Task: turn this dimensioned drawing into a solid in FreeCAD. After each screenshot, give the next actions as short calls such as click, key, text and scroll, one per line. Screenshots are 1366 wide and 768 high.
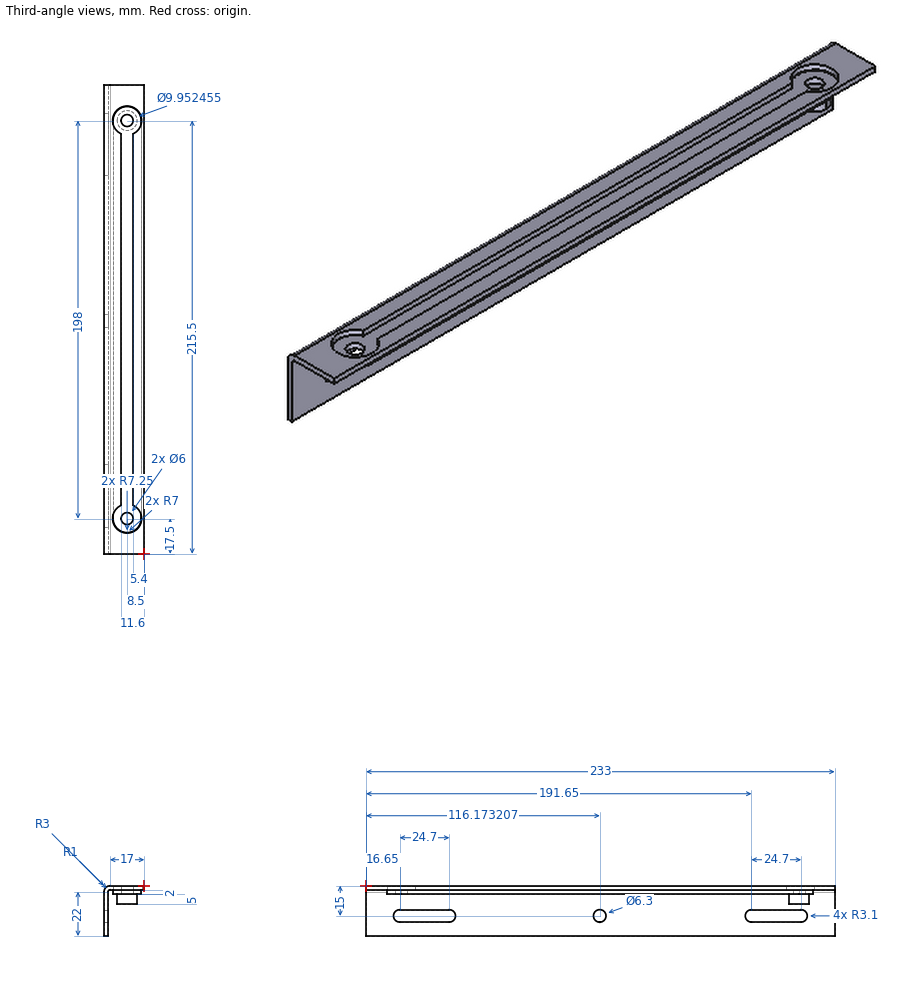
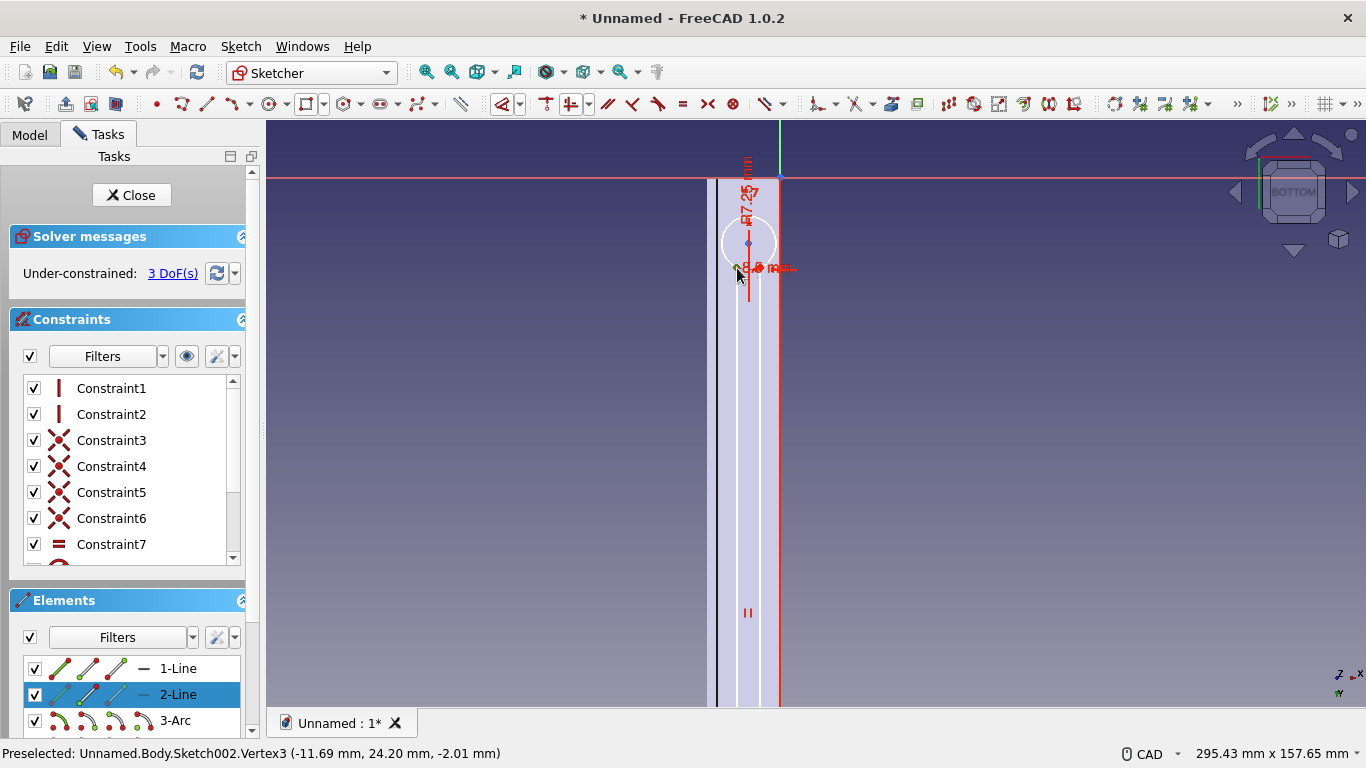
click(520, 104)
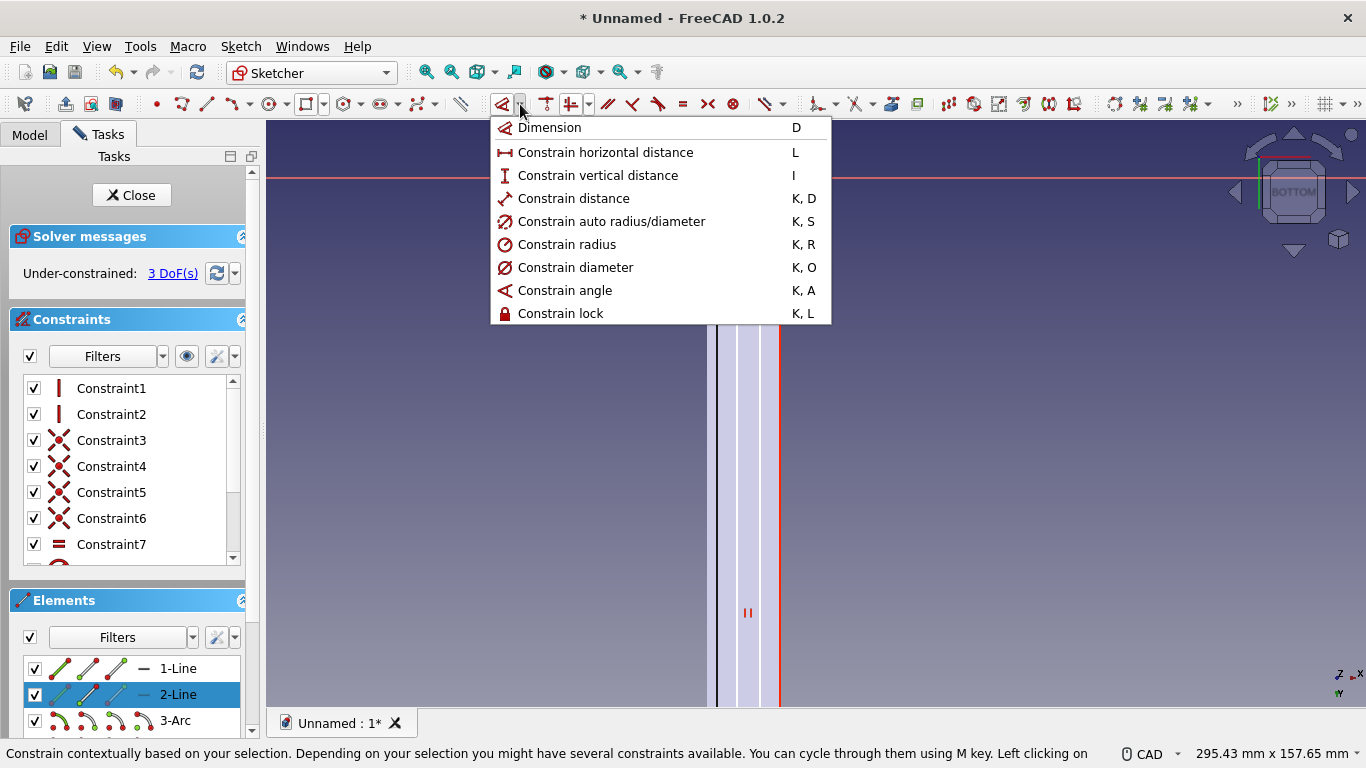
click(661, 152)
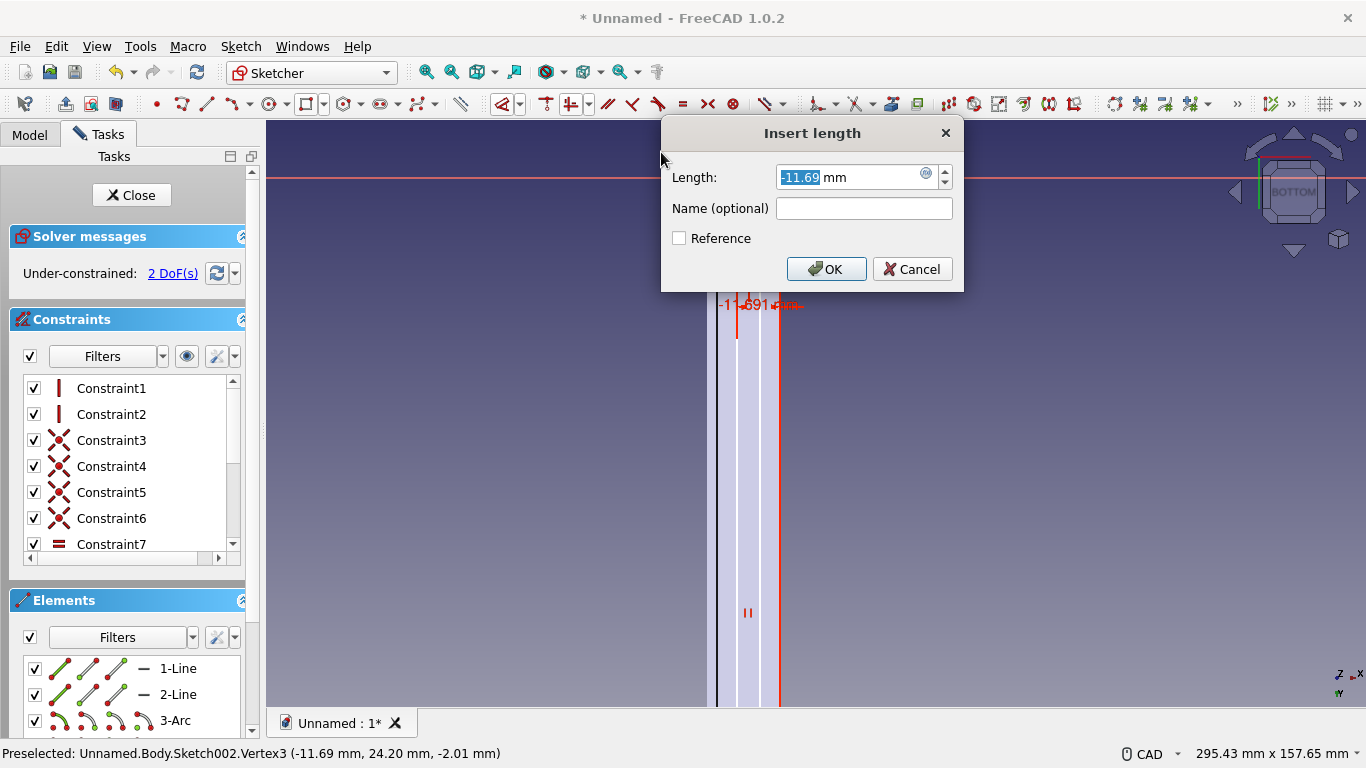
text(-11.6)
key(Return)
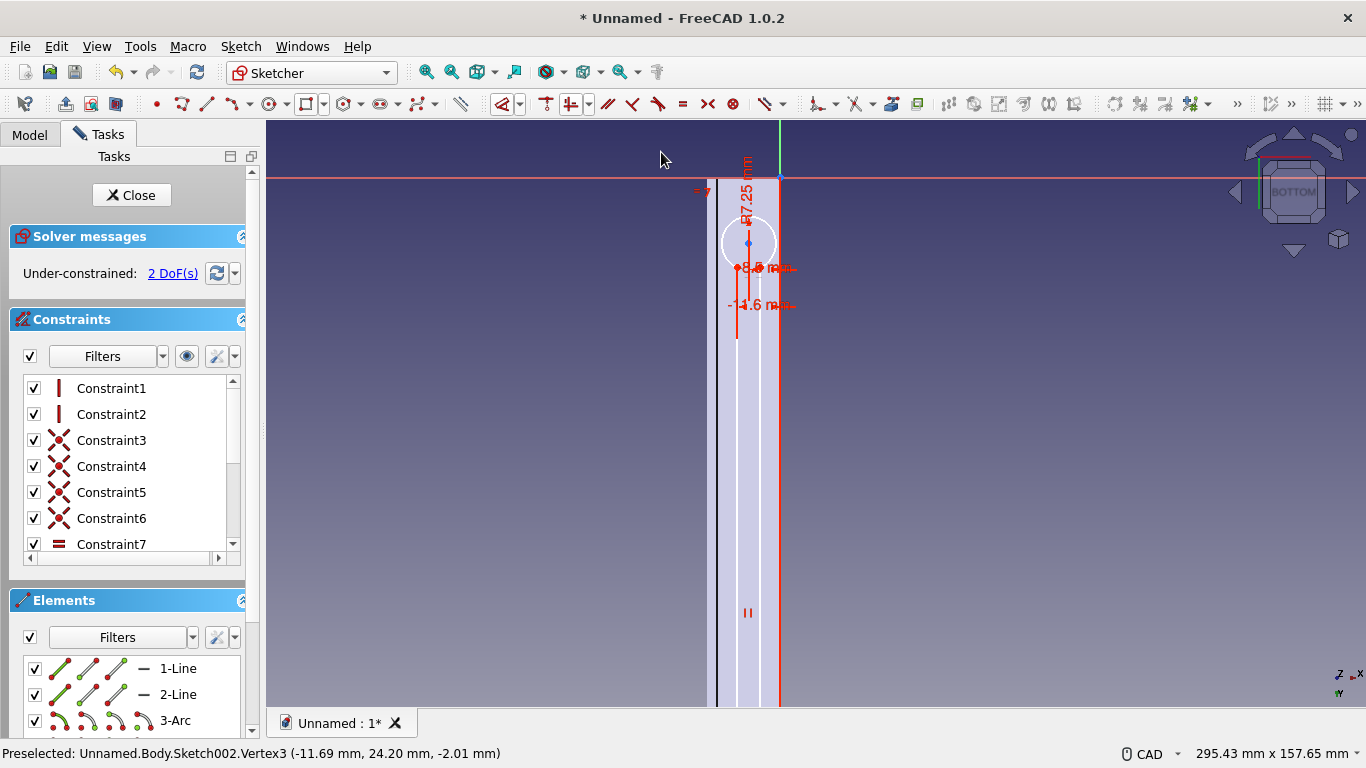
click(749, 243)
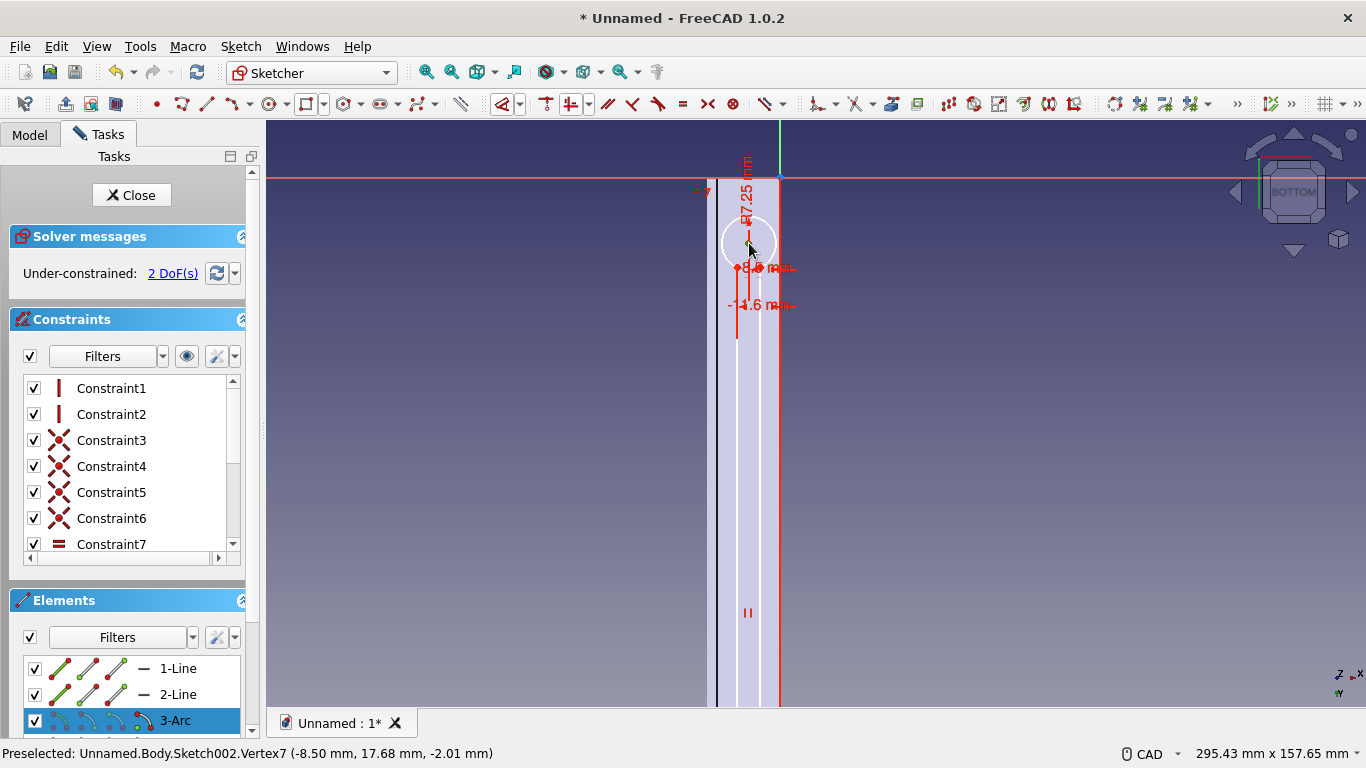
click(520, 104)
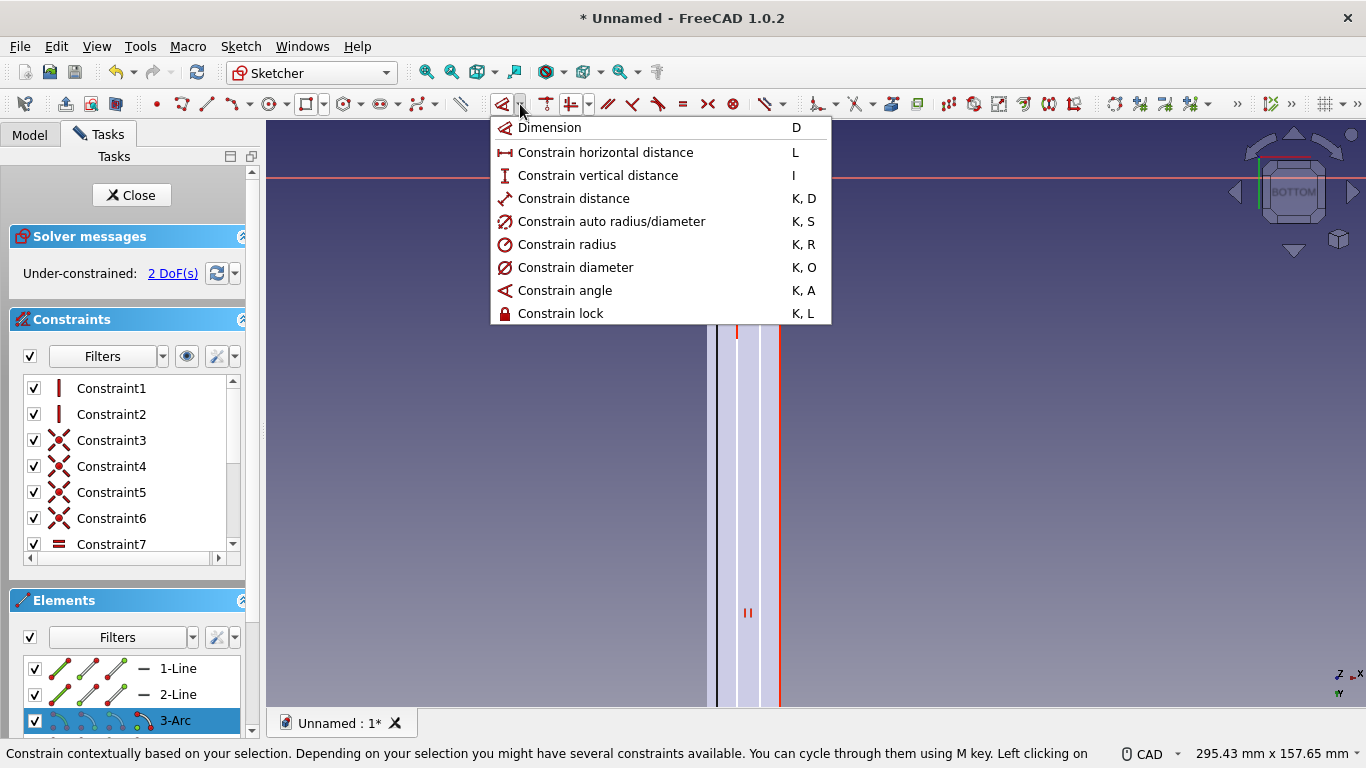
click(661, 176)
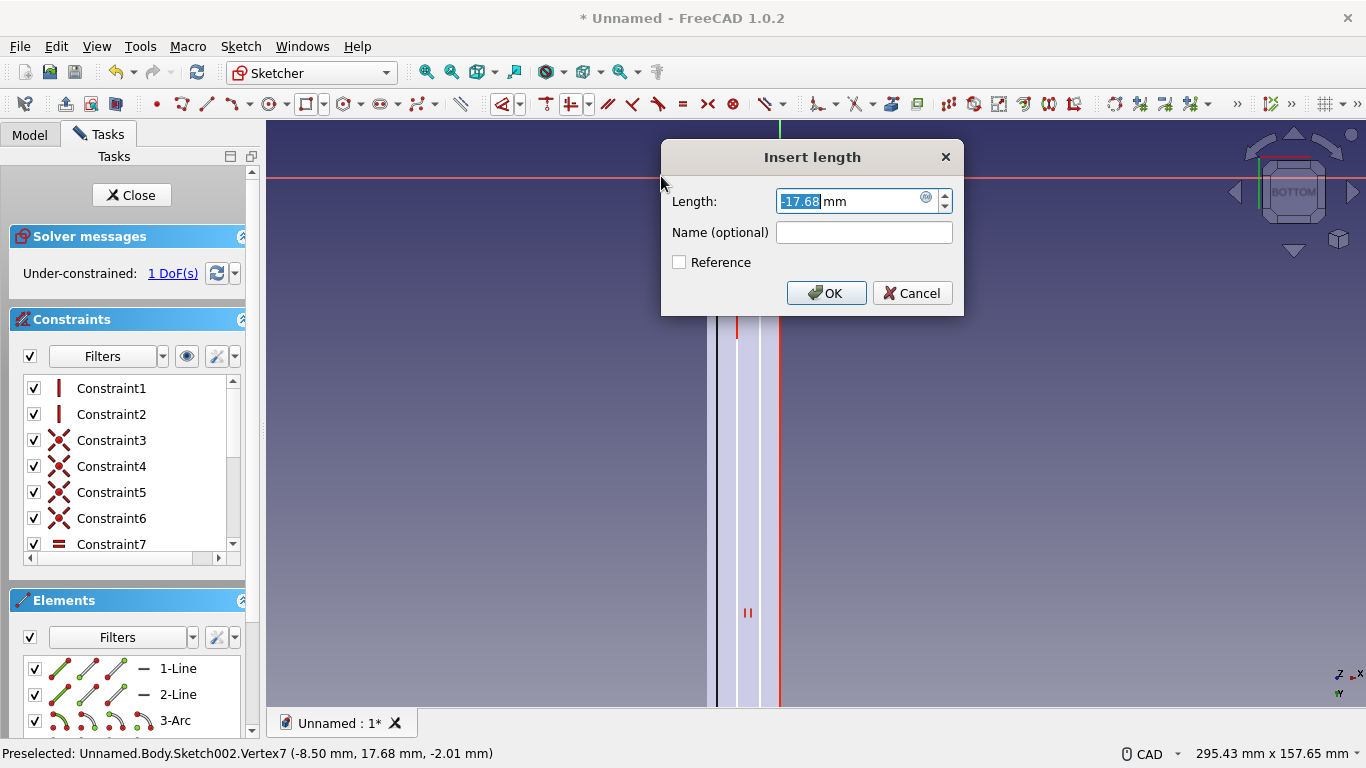
text(-17.5)
key(Return)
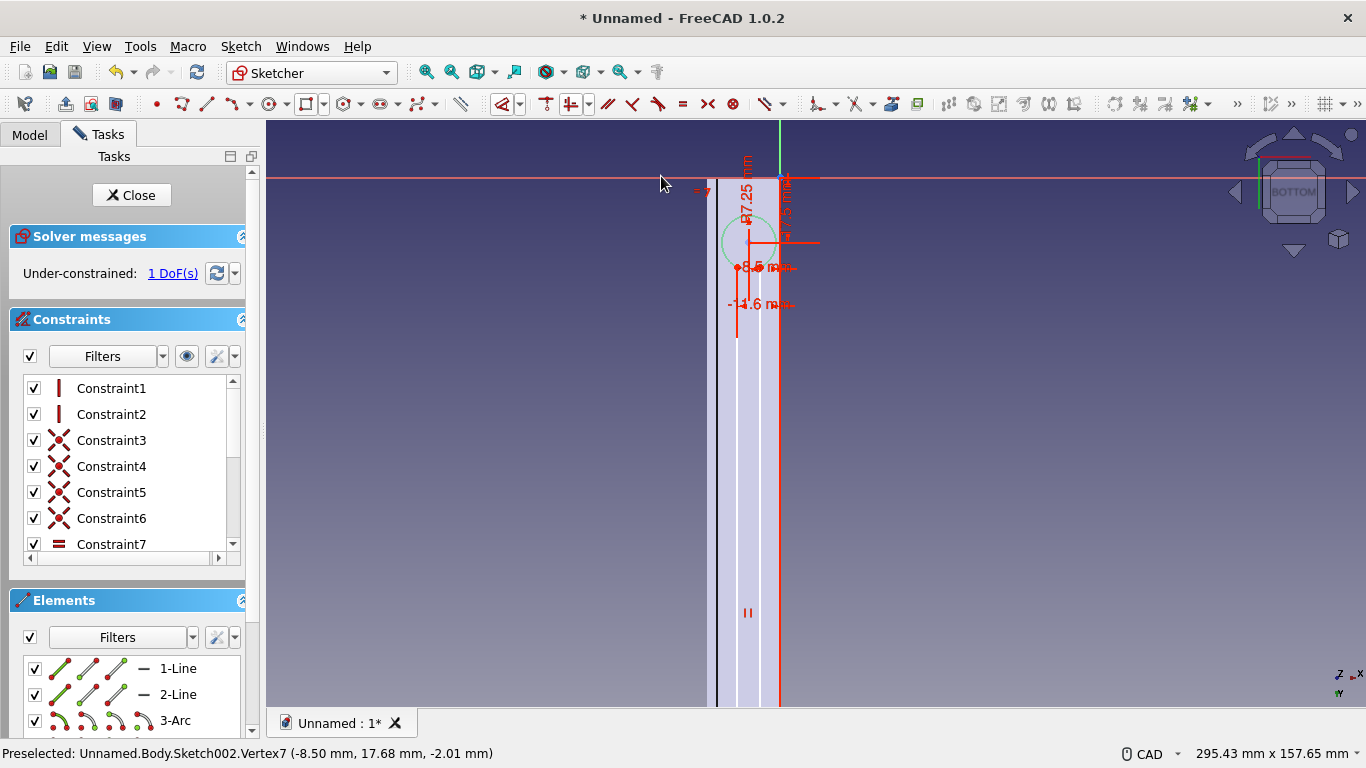
scroll(738, 268, down, 4)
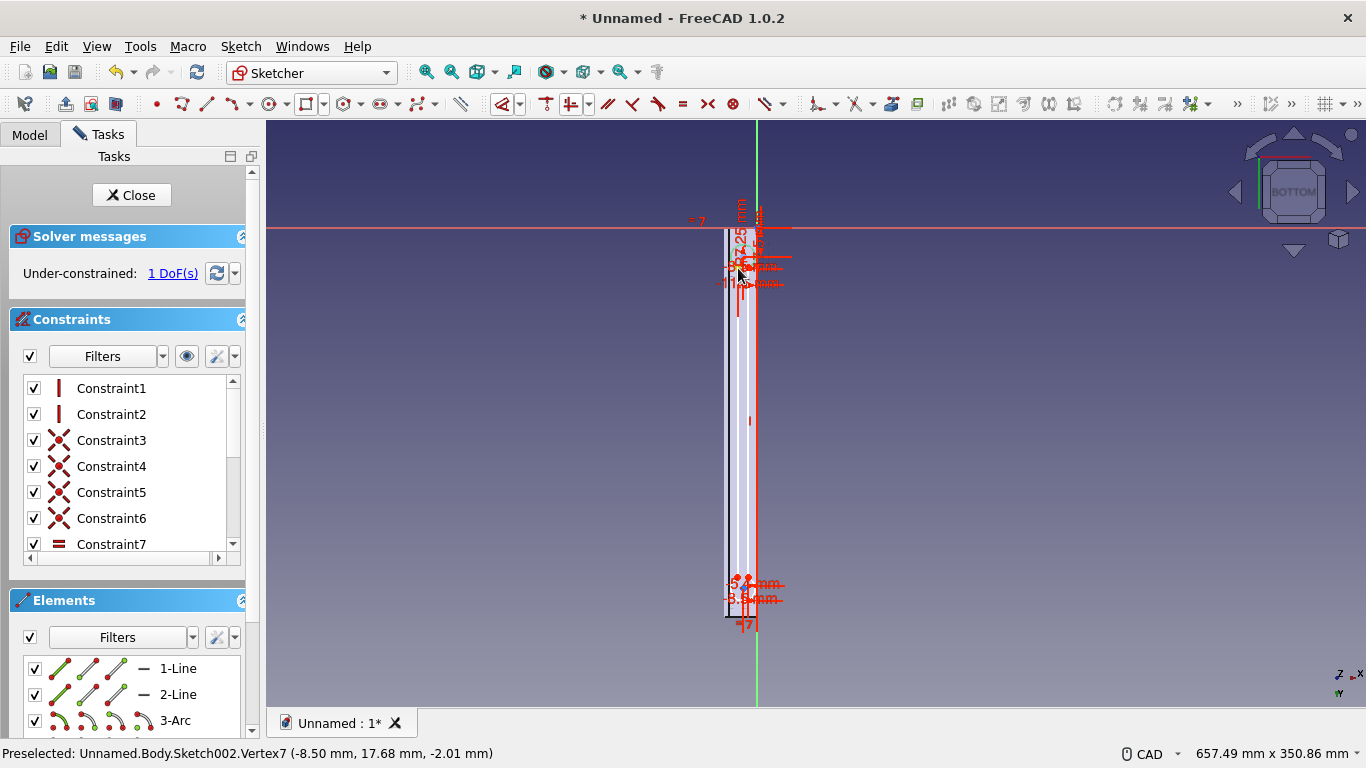
click(743, 589)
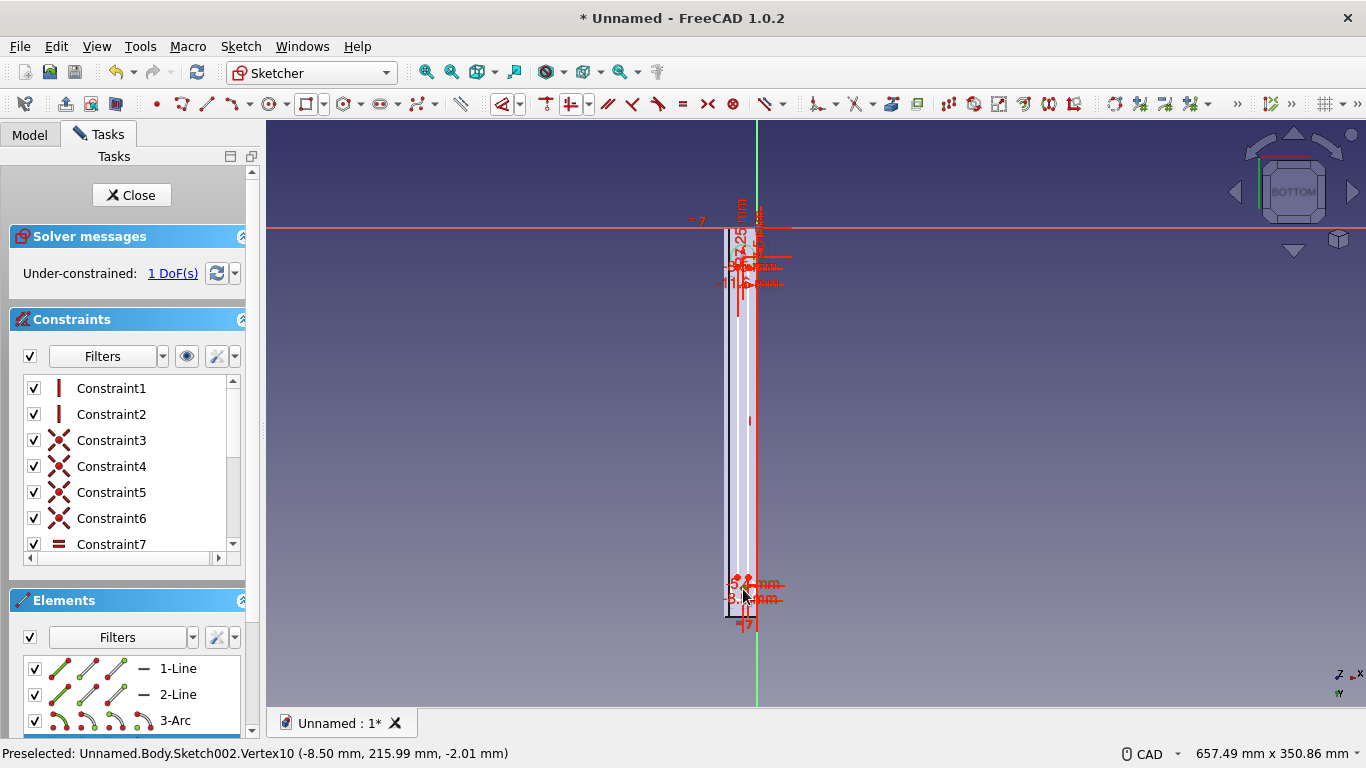
click(520, 104)